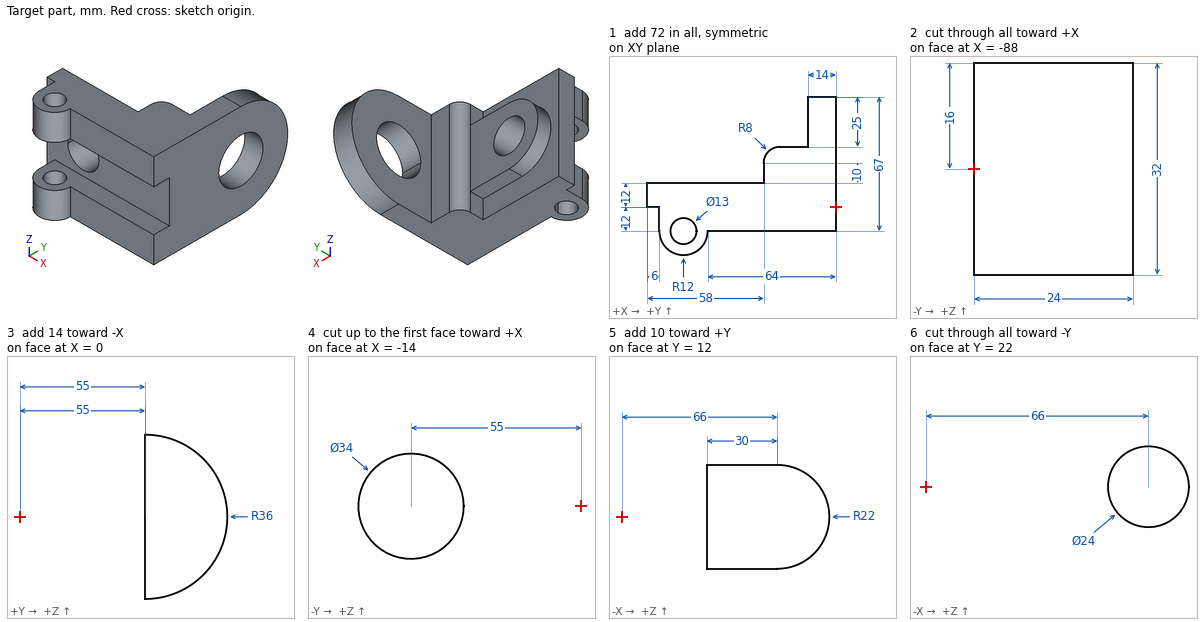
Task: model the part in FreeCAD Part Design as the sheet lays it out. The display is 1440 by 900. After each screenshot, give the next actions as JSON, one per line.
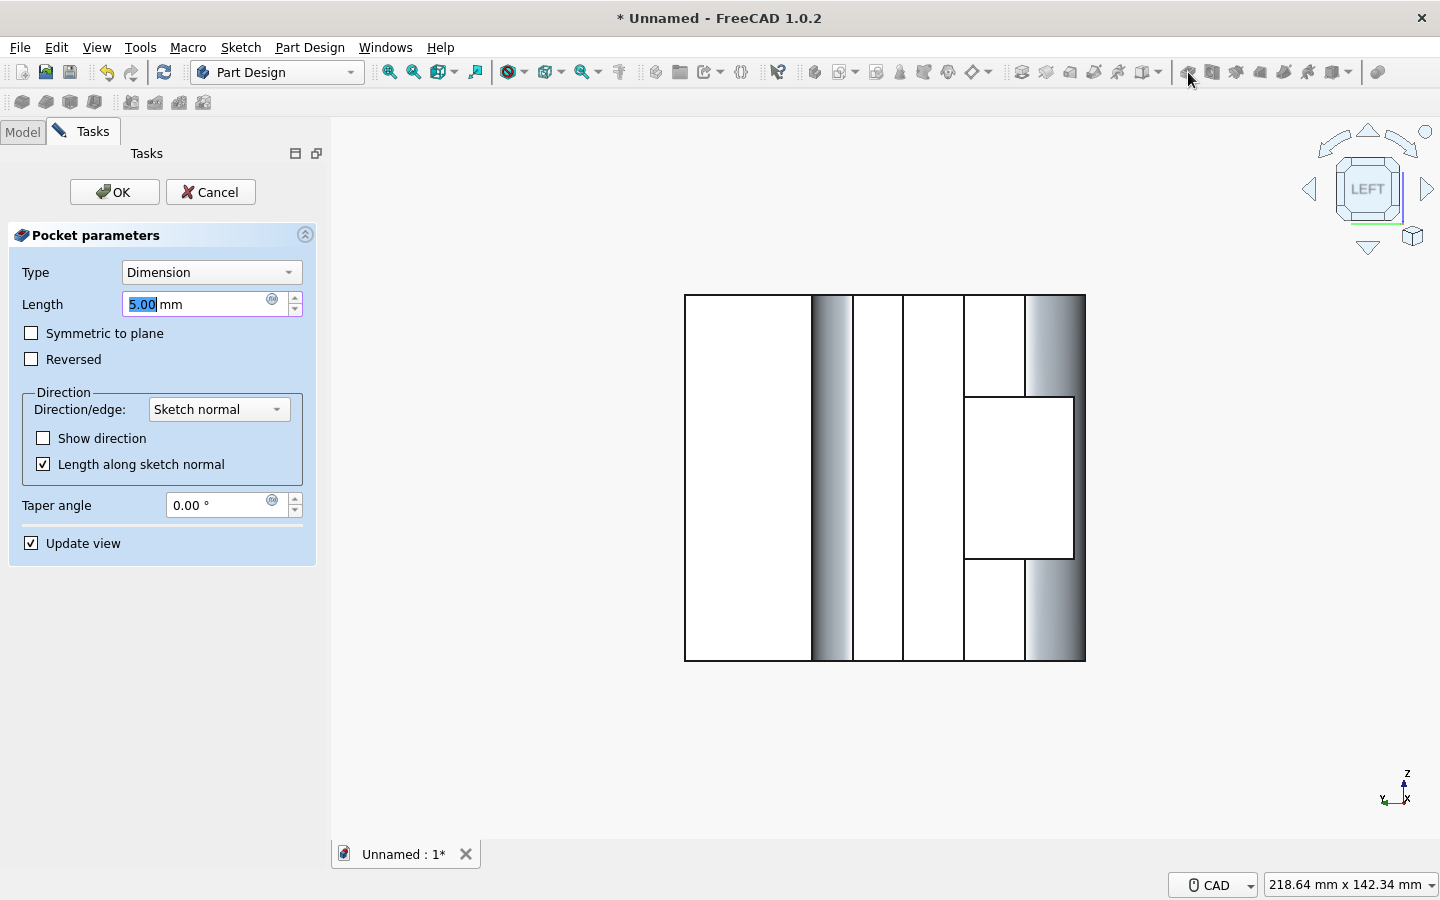
{"action": "left_click", "coordinate": [212, 272]}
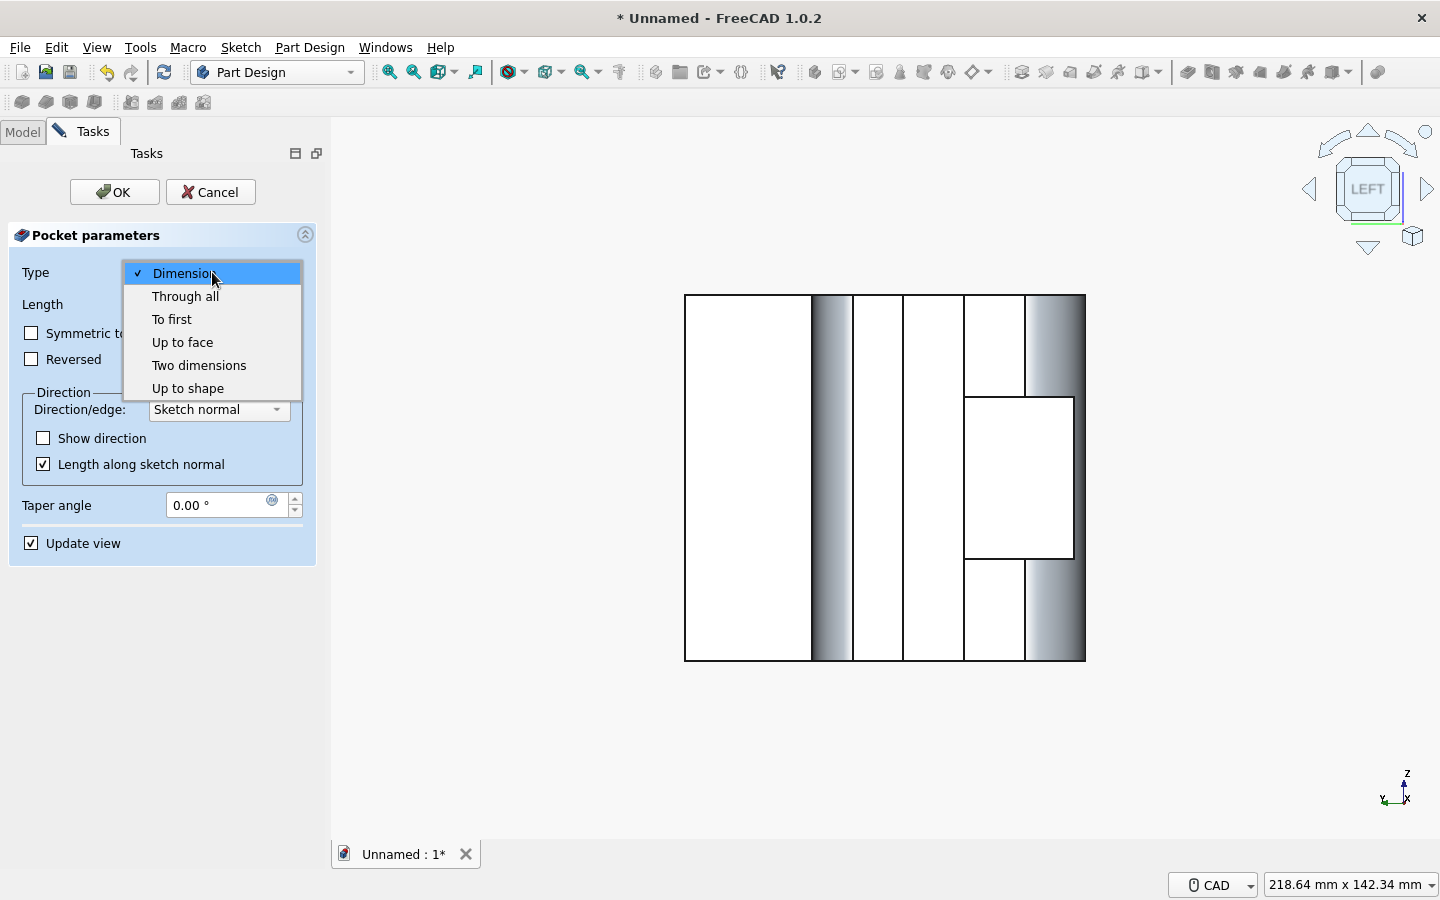
{"action": "left_click", "coordinate": [212, 296]}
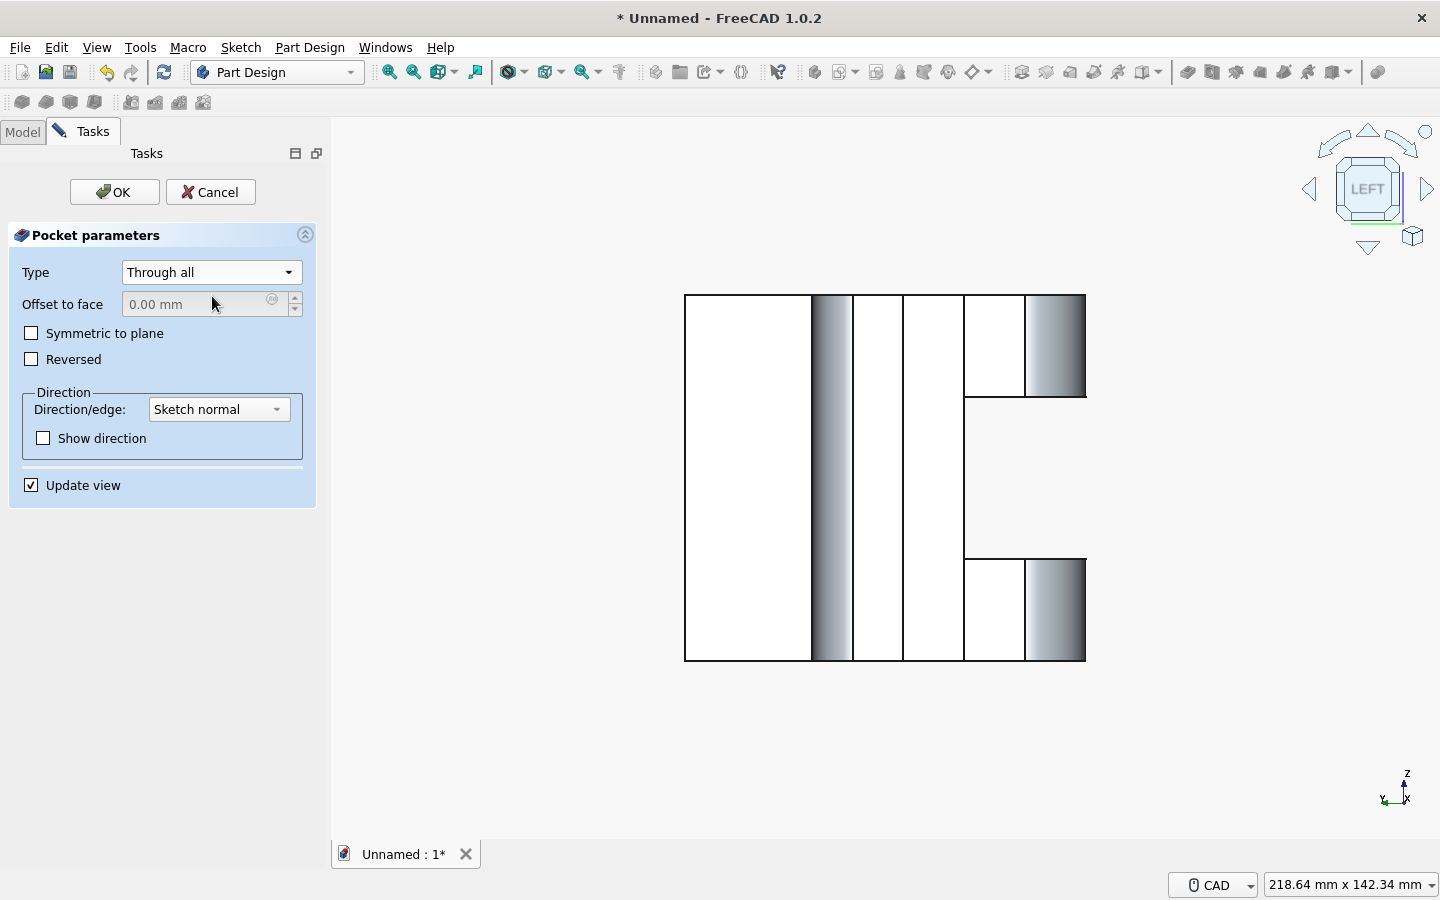
{"action": "left_click", "coordinate": [115, 192]}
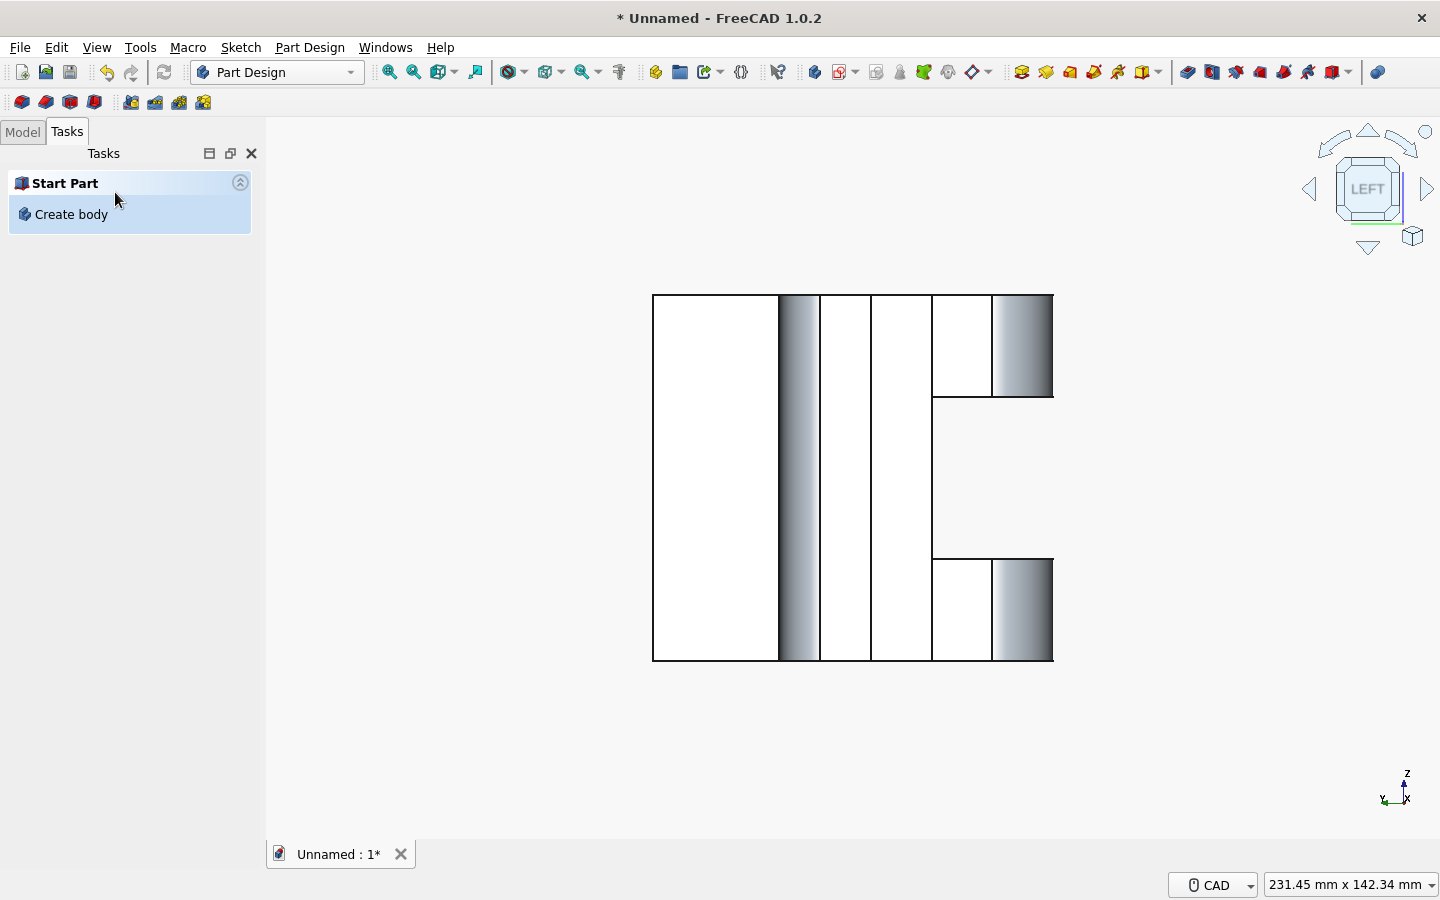
{"action": "key", "text": "0"}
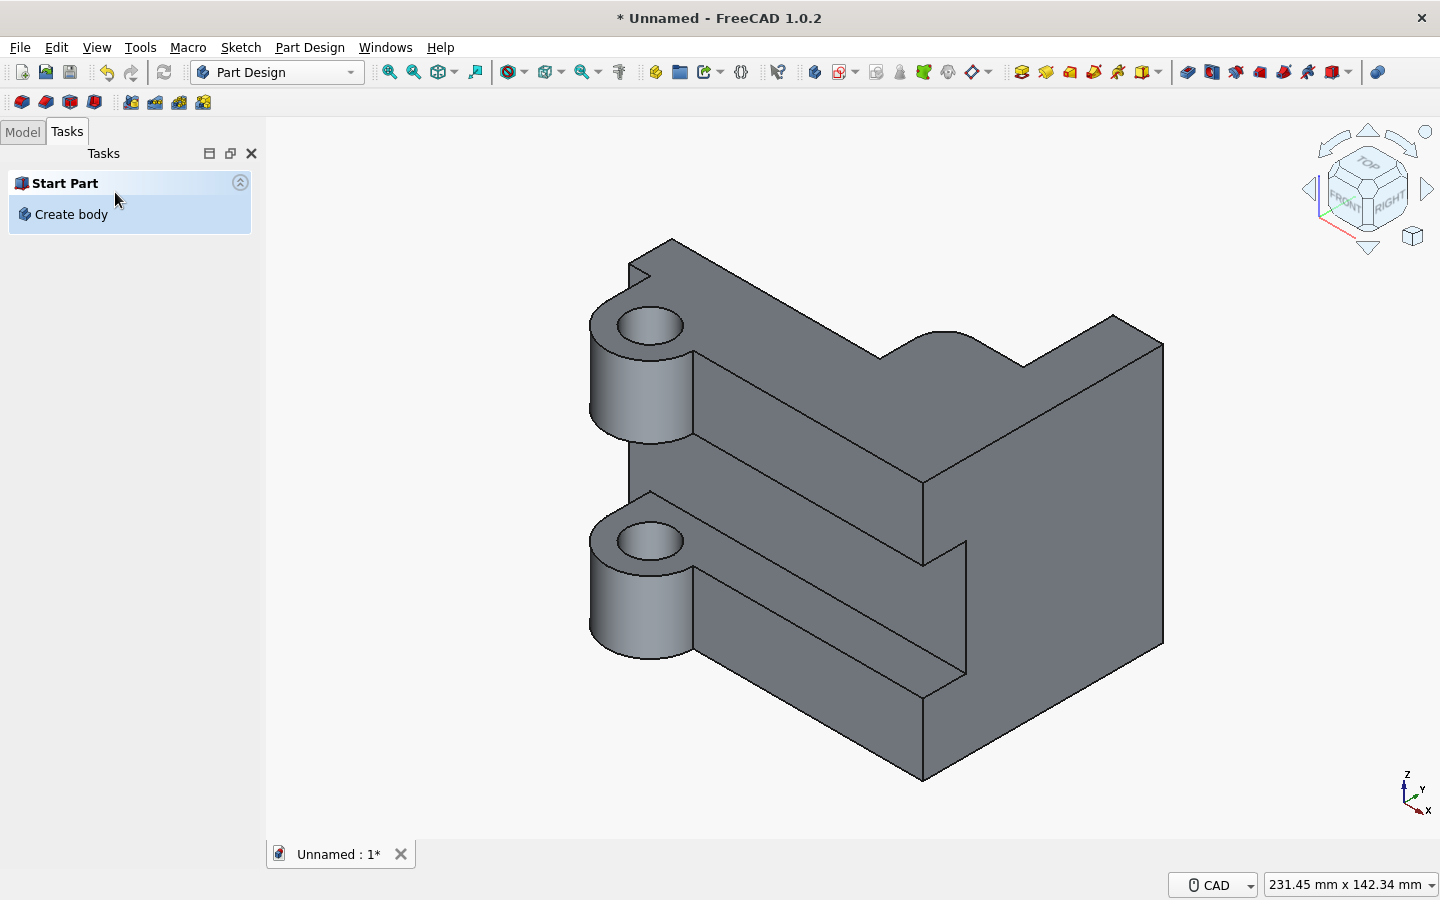
{"action": "left_click", "coordinate": [1077, 499]}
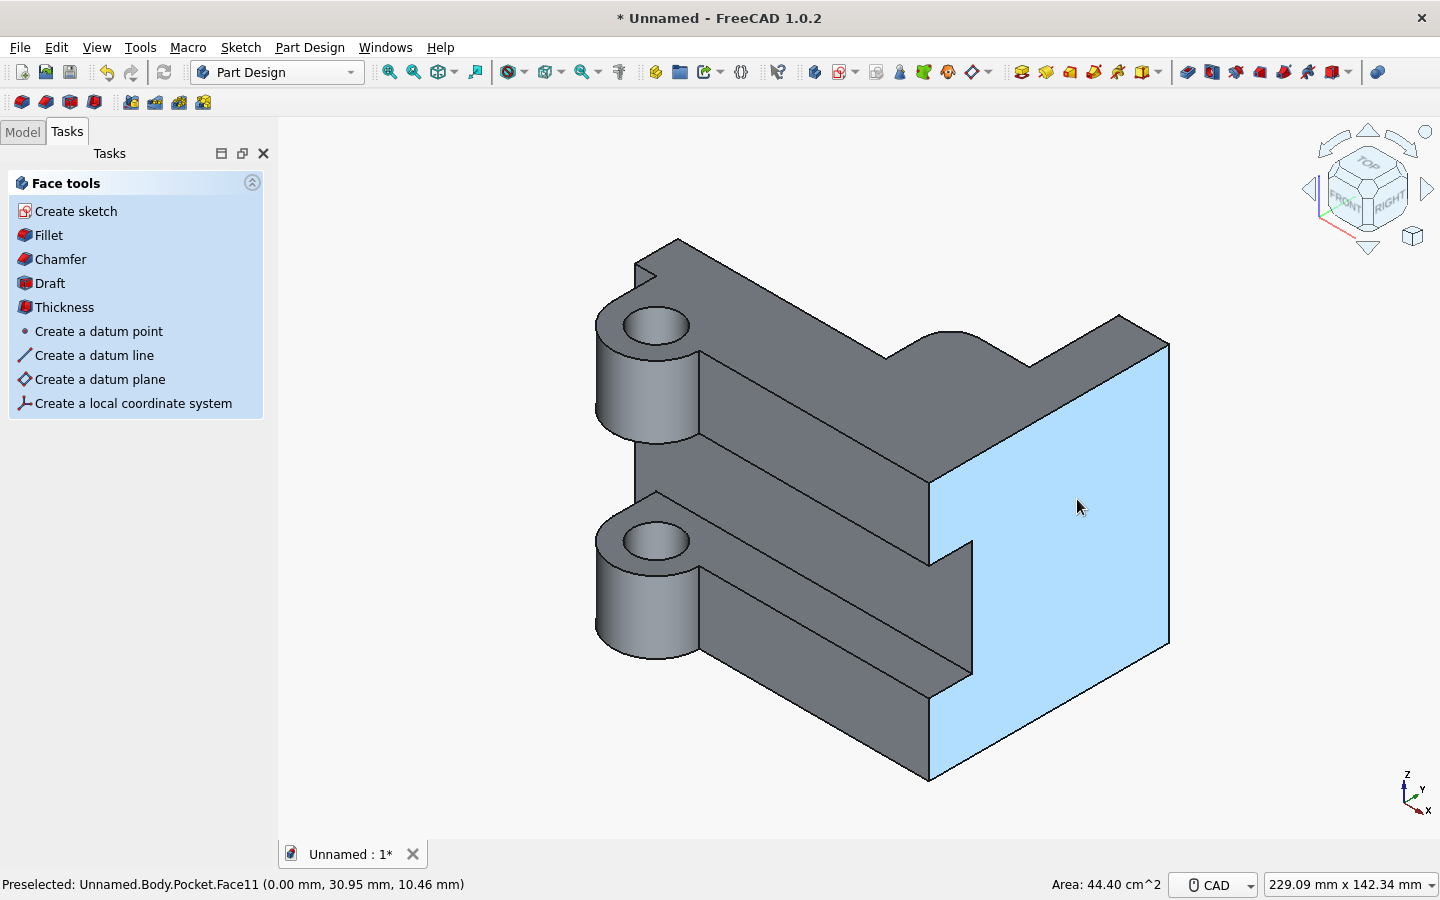
{"action": "left_click", "coordinate": [840, 72]}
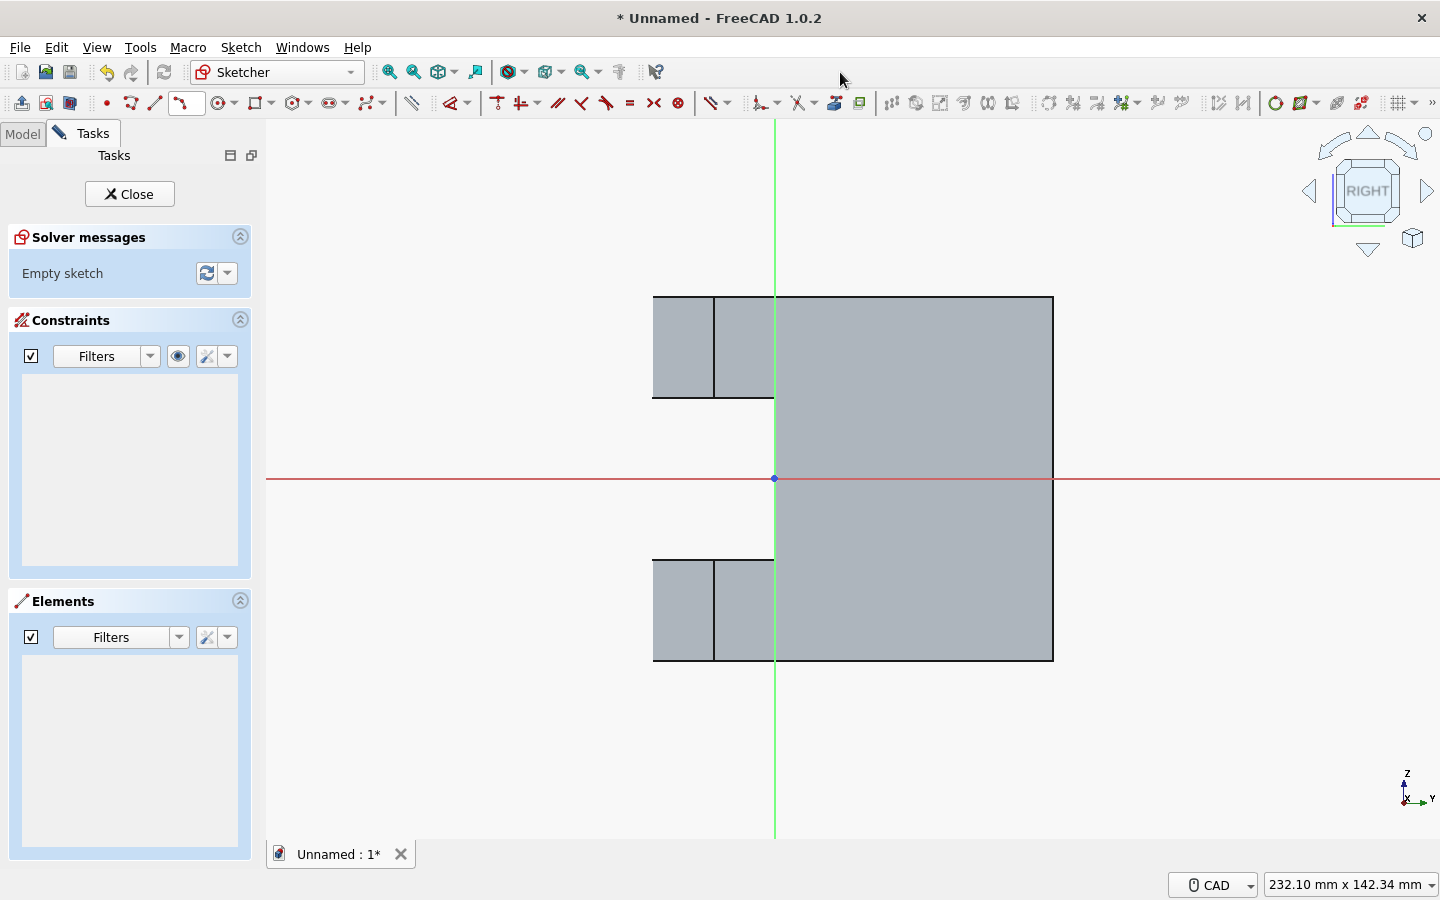
{"action": "left_click", "coordinate": [156, 104]}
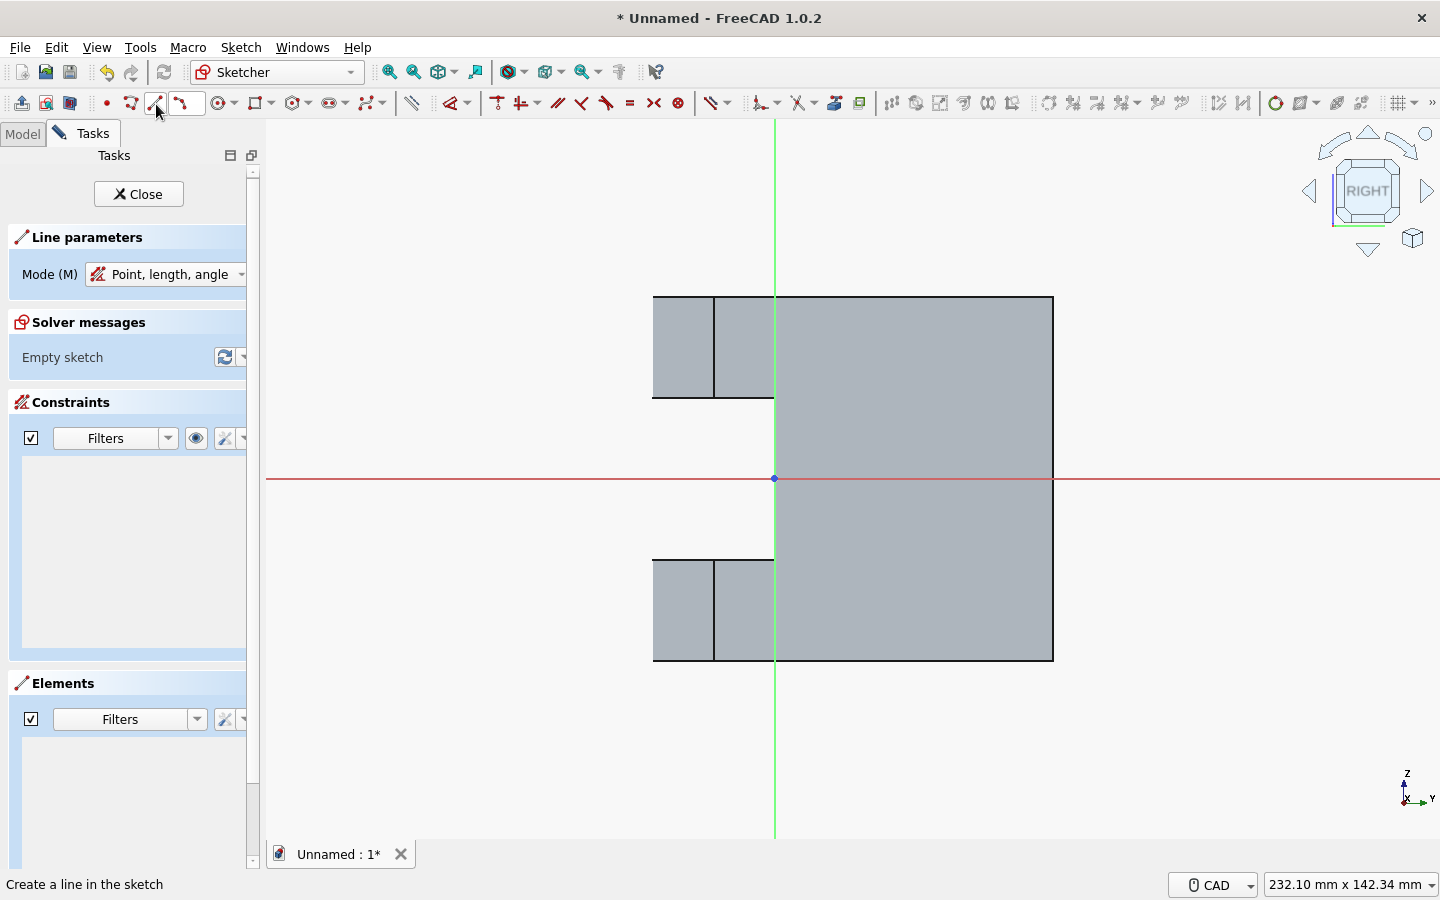
{"action": "left_click", "coordinate": [1053, 297]}
{"action": "left_click", "coordinate": [1053, 661]}